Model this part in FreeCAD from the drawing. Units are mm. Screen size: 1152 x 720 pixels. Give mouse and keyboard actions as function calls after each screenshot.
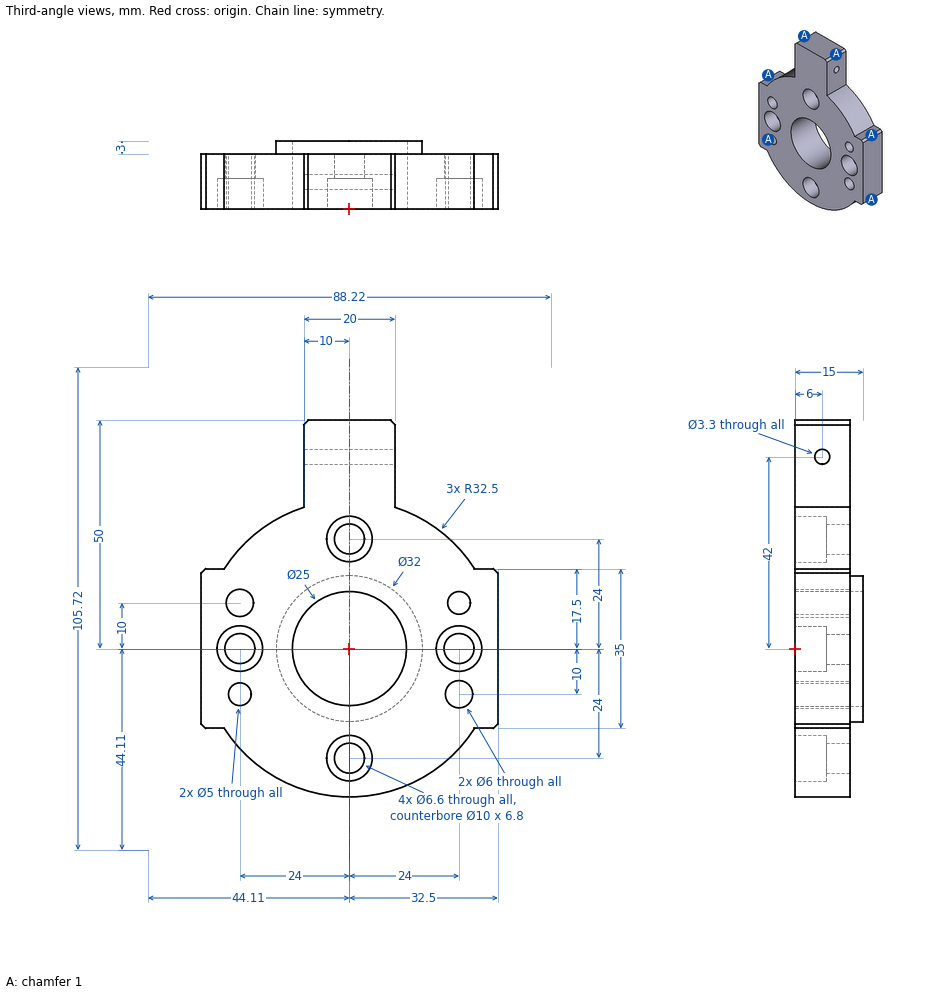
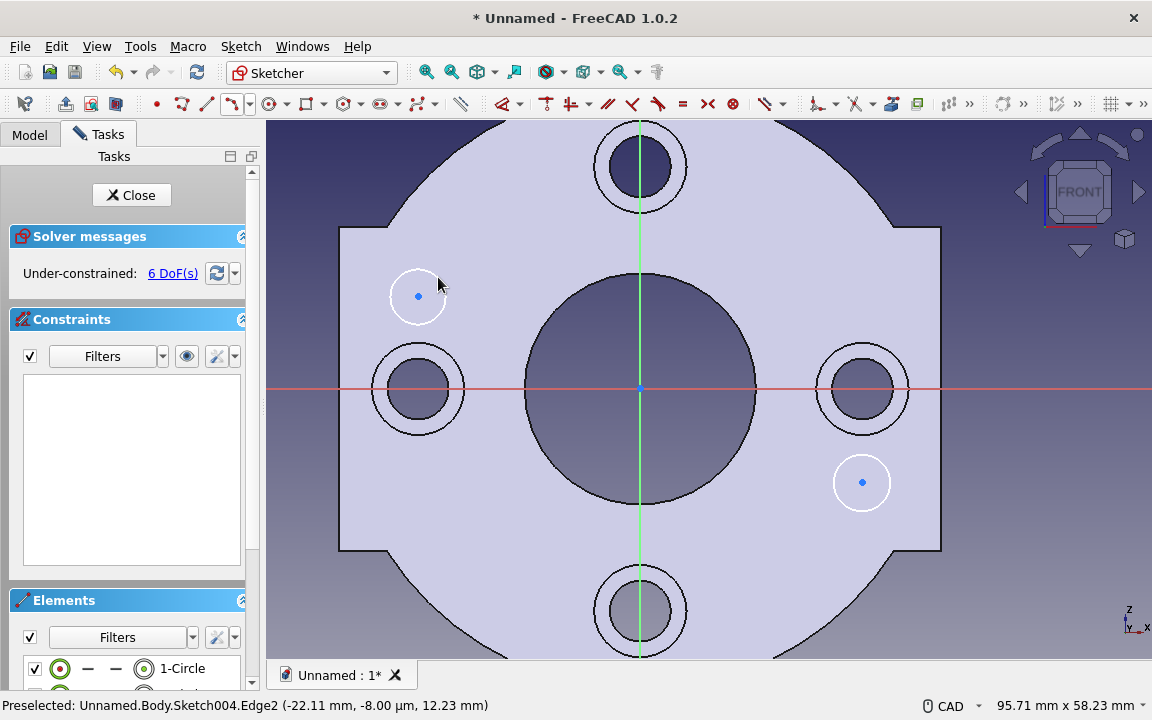
click(882, 463)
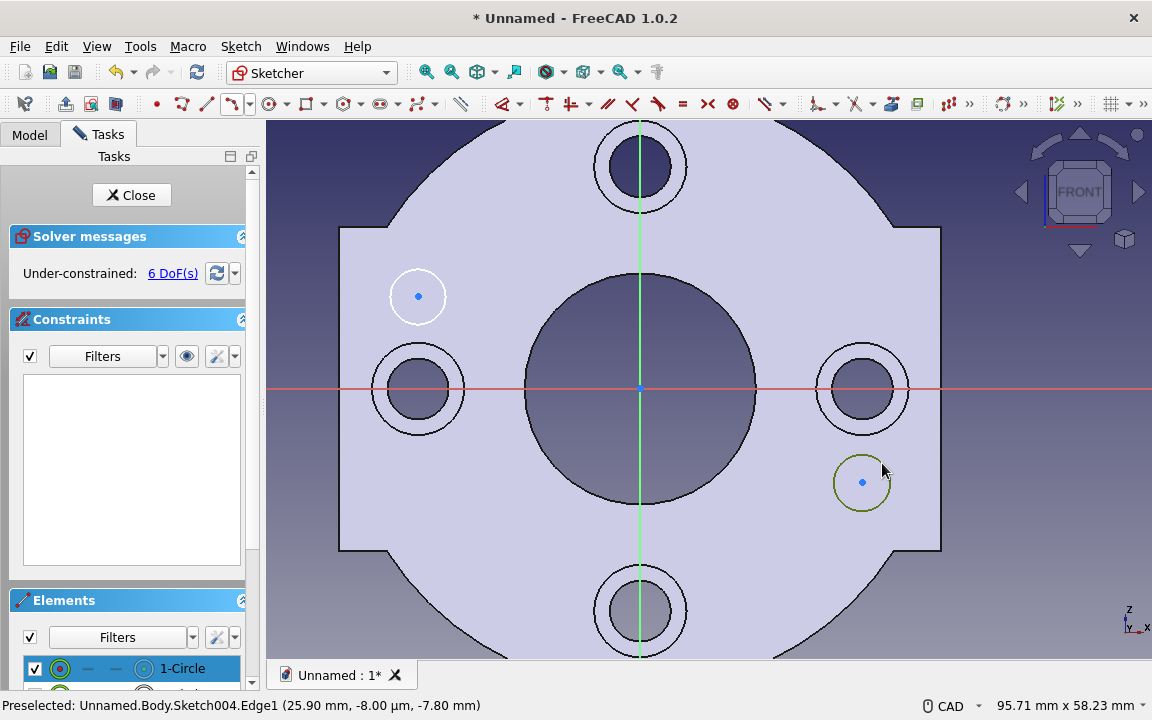
click(437, 277)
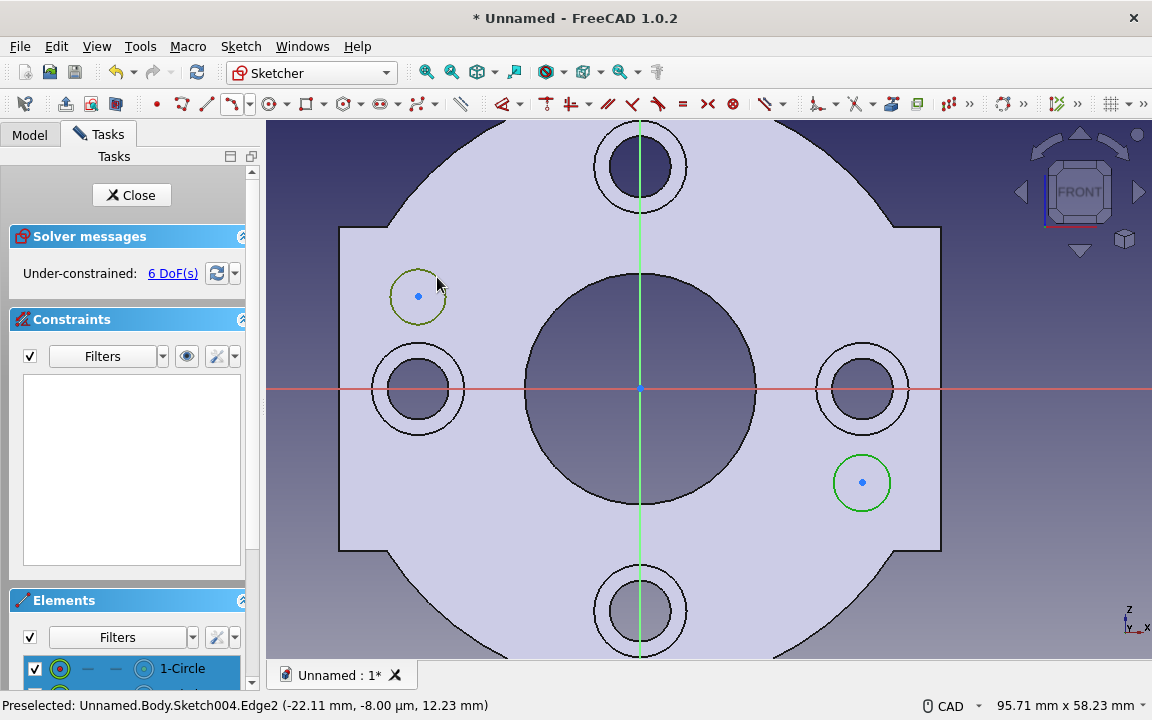
click(683, 104)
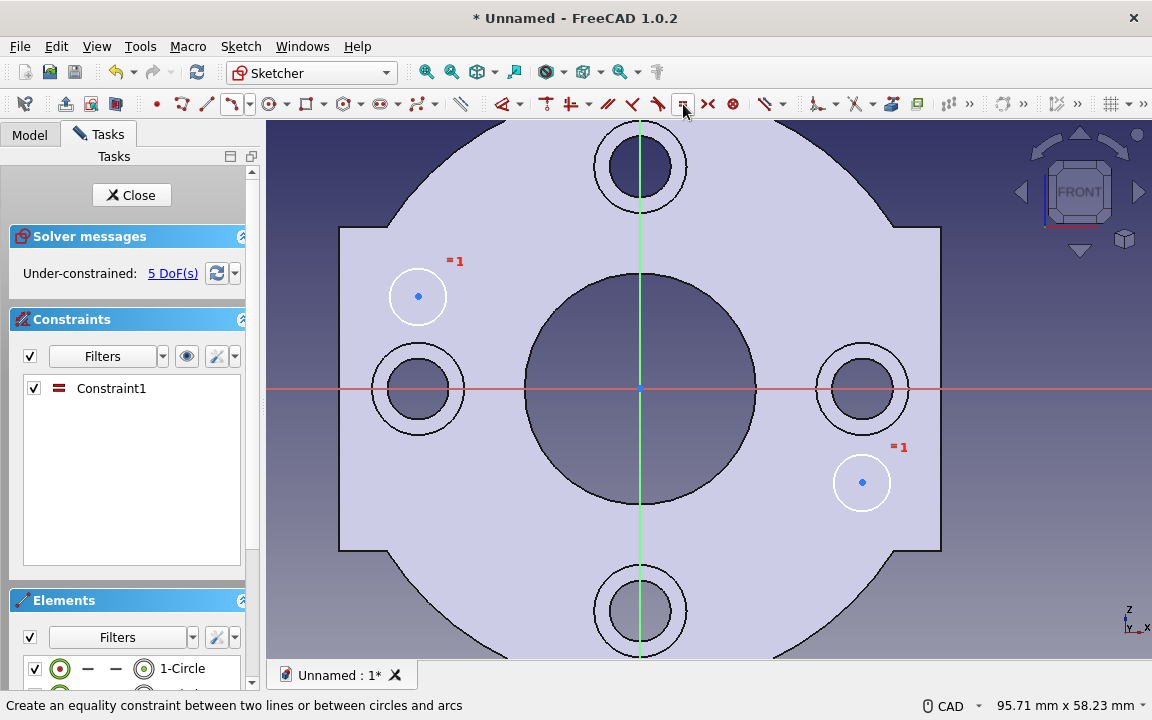
click(502, 104)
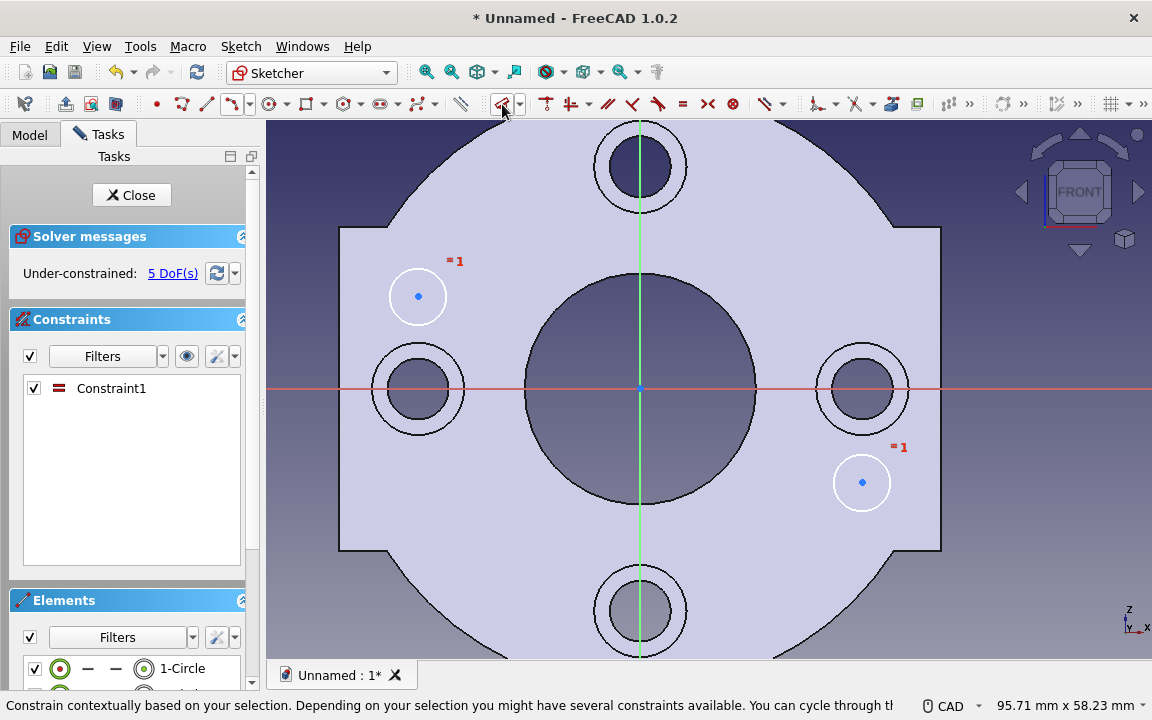
click(882, 463)
click(905, 440)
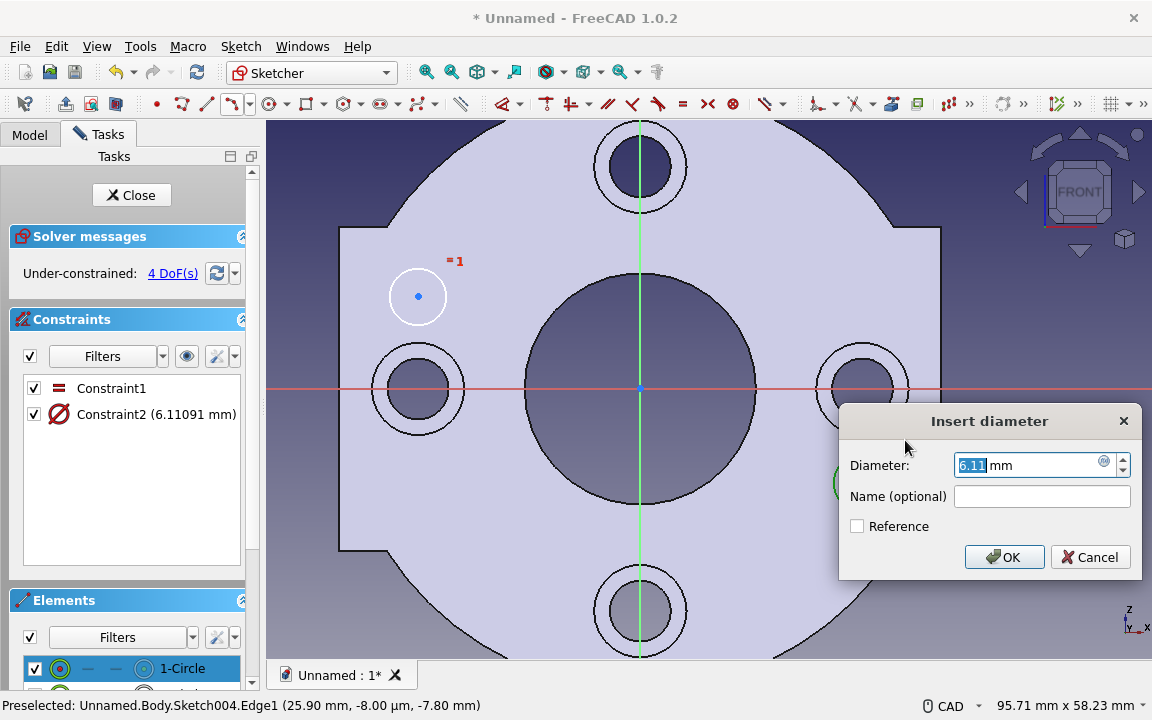
text(6)
key(Return)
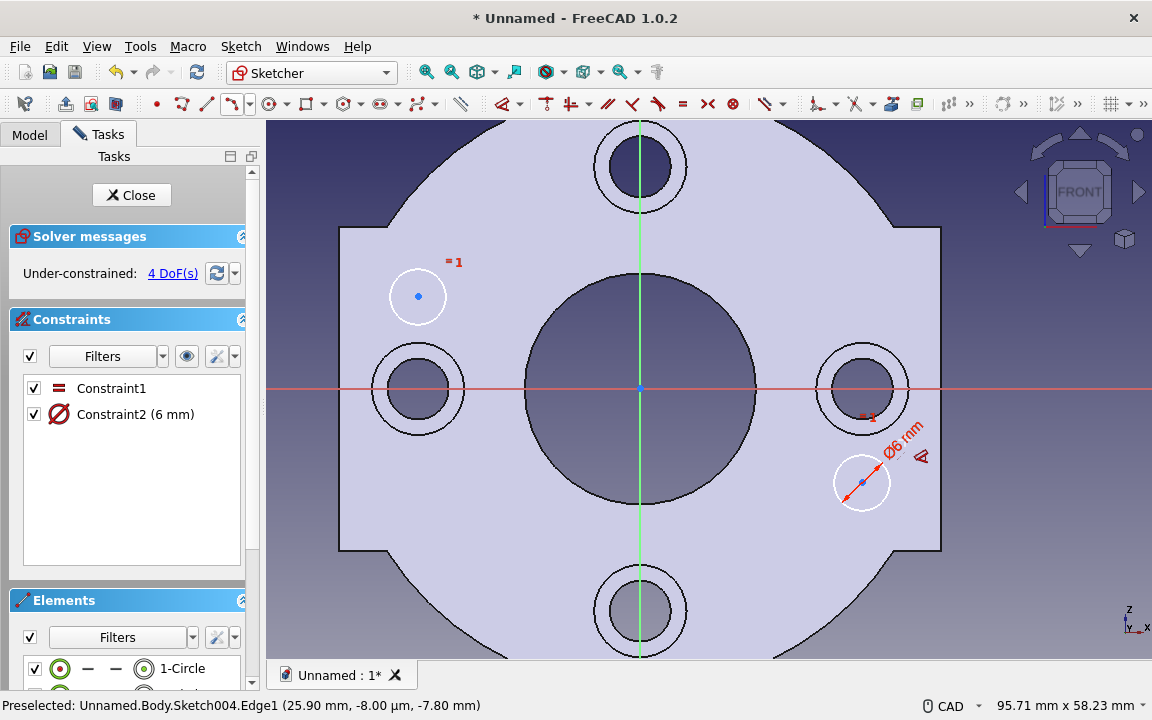
click(862, 483)
click(751, 517)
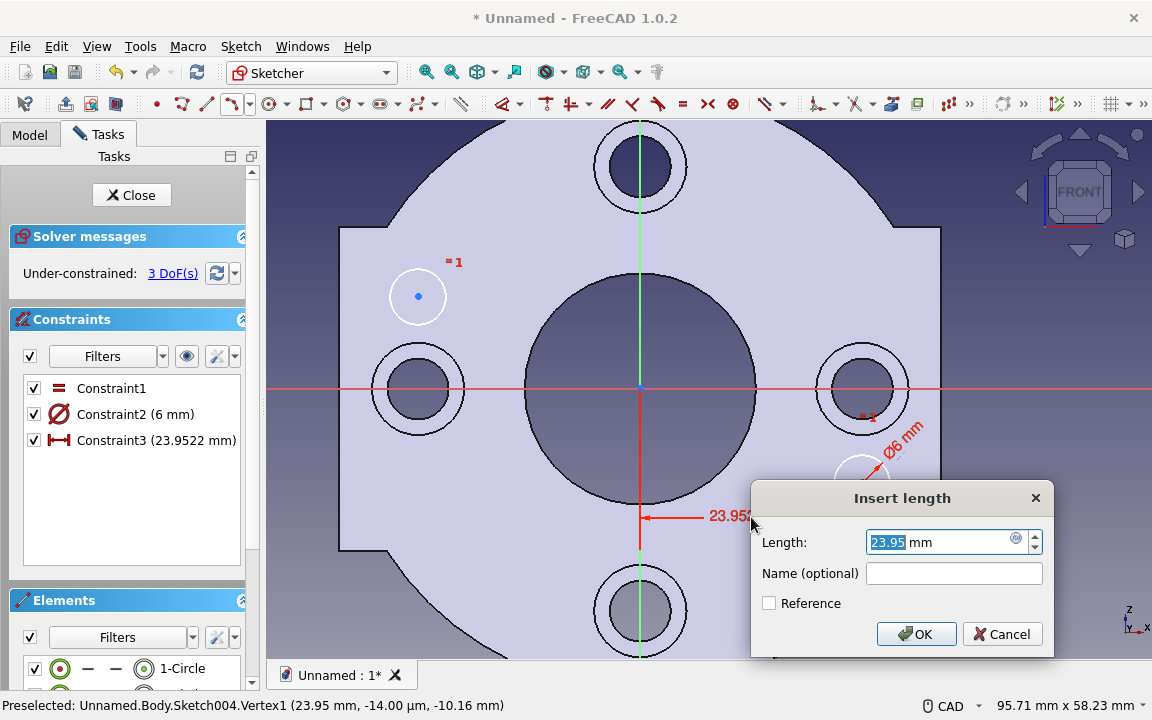
text(24)
key(Return)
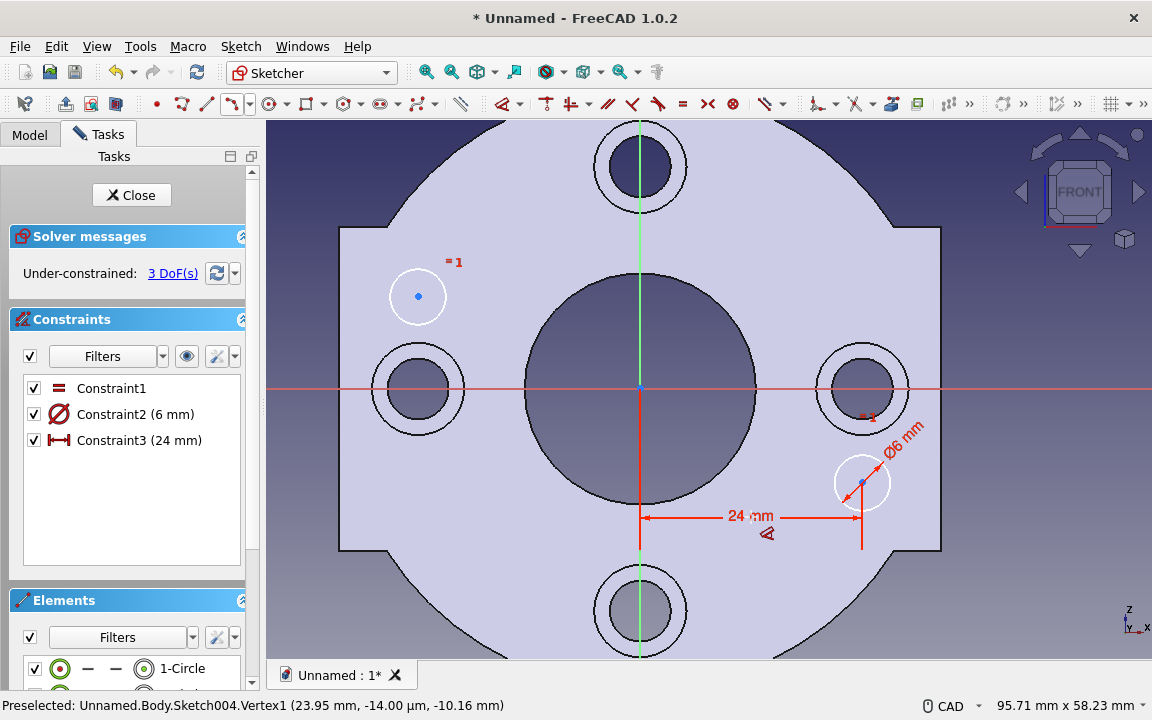
click(862, 483)
click(896, 414)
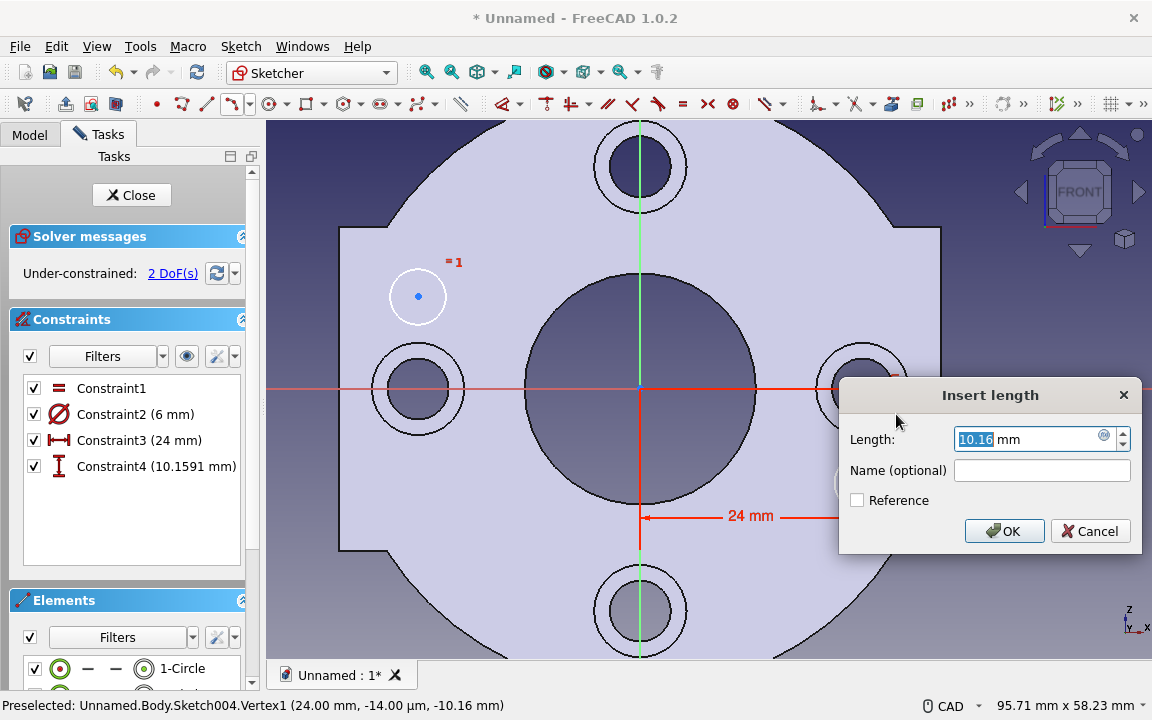
text(10)
key(Return)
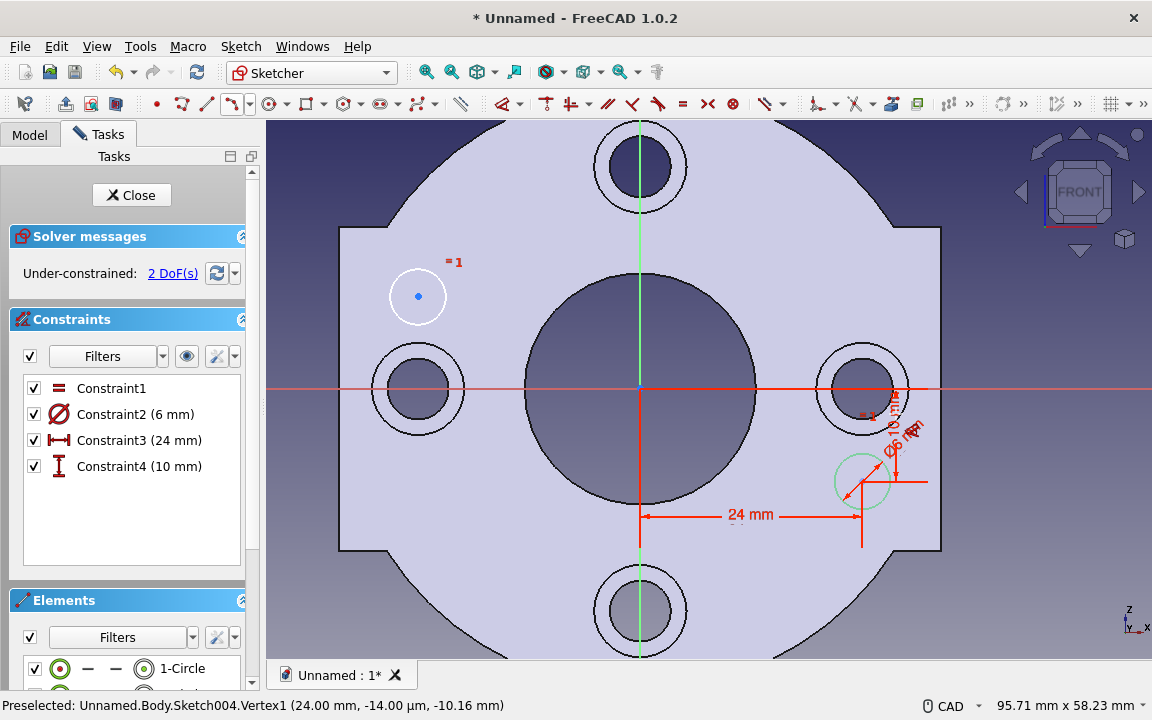
click(418, 297)
click(529, 263)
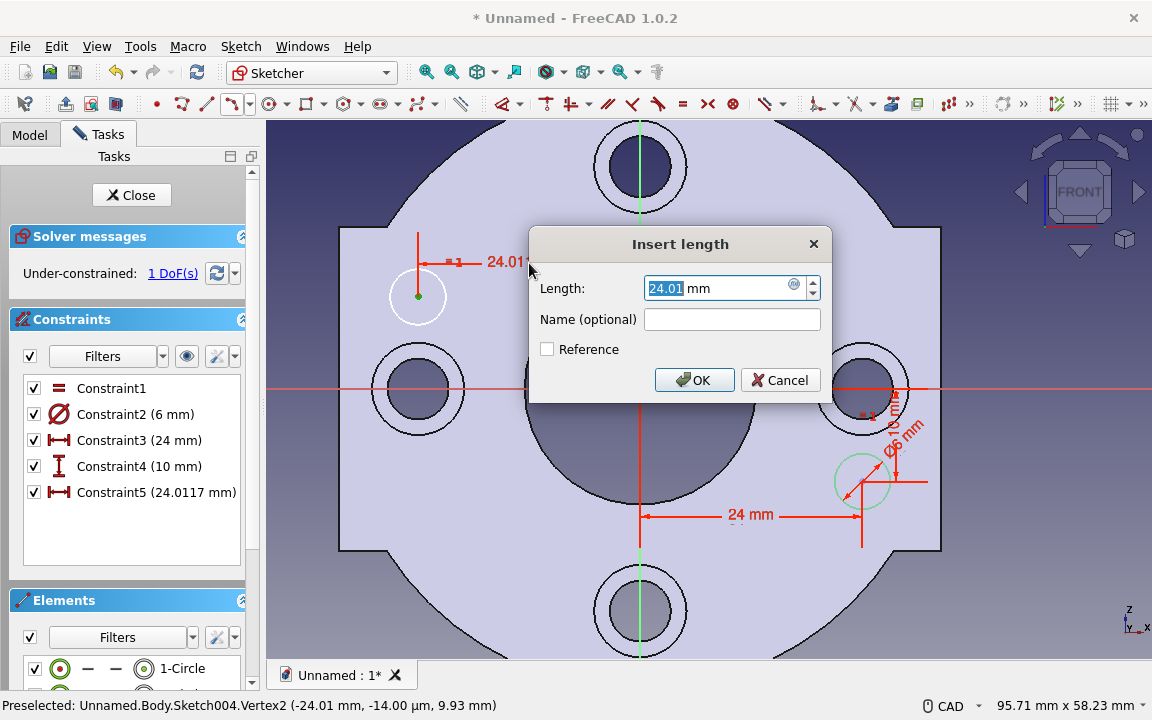
text(24)
key(Return)